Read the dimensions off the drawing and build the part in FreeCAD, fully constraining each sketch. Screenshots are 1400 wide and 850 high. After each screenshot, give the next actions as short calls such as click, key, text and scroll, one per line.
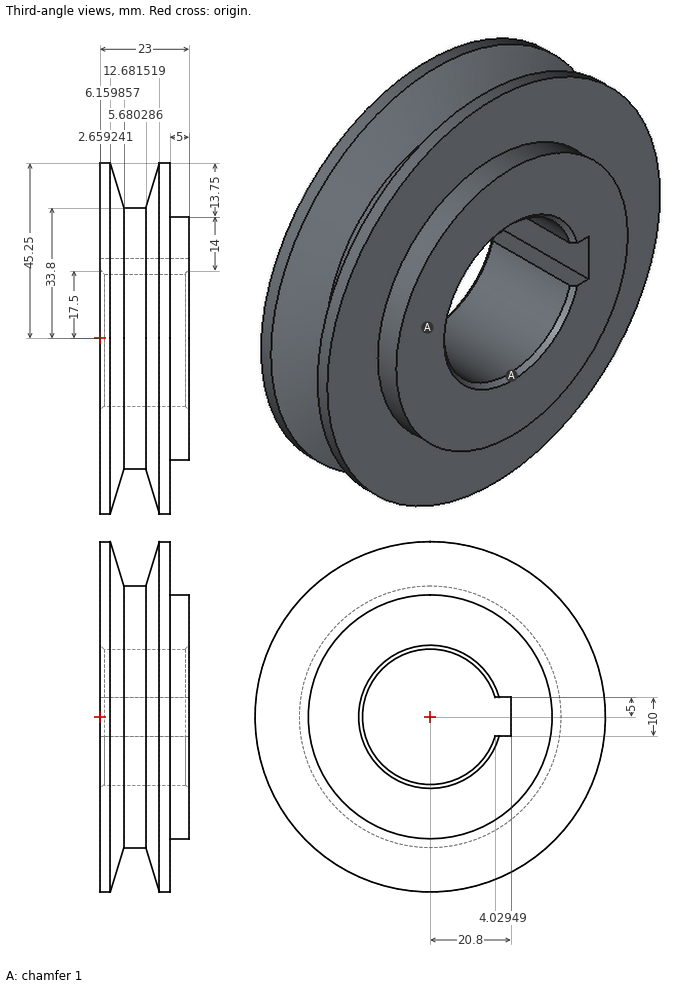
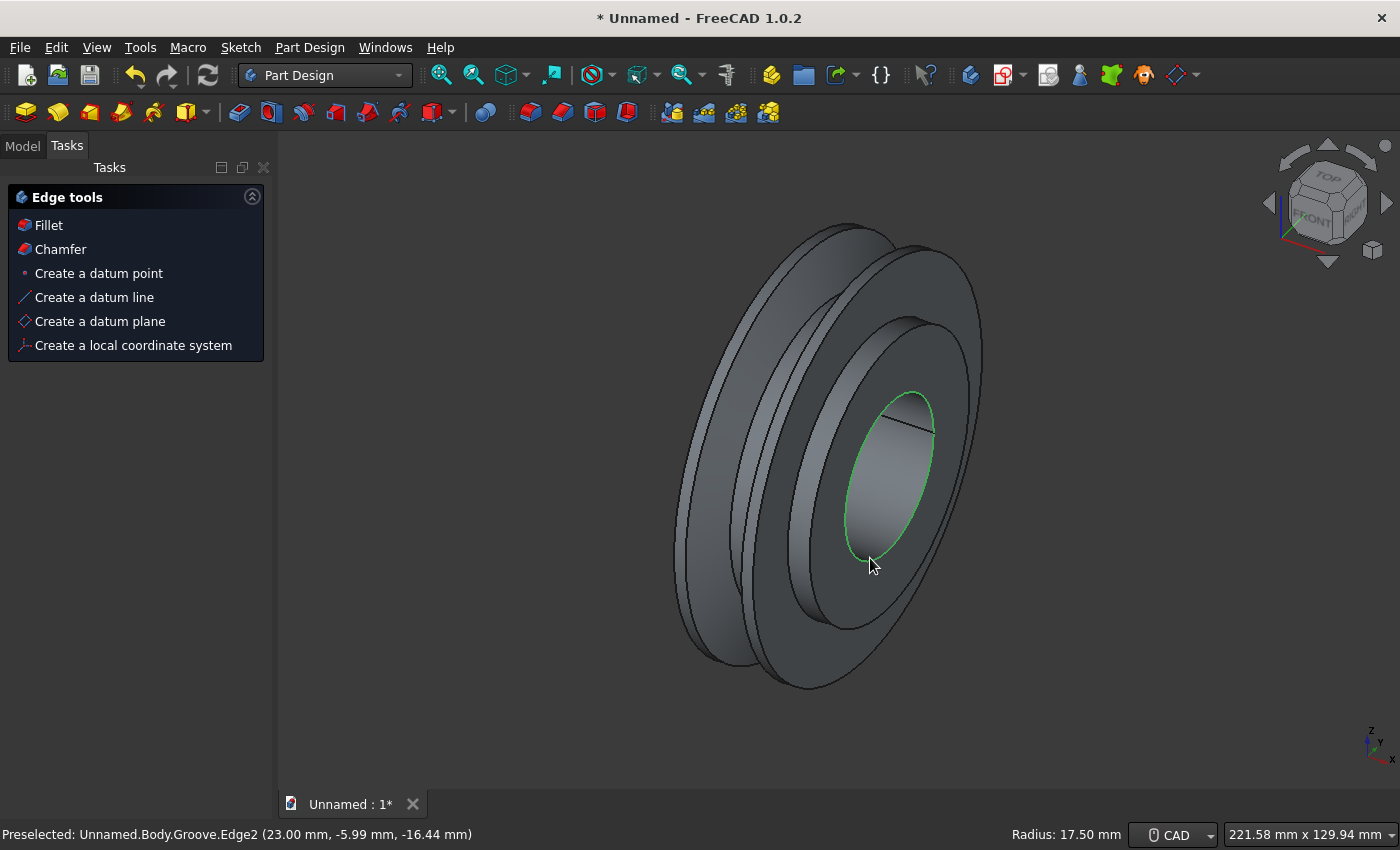
key(0)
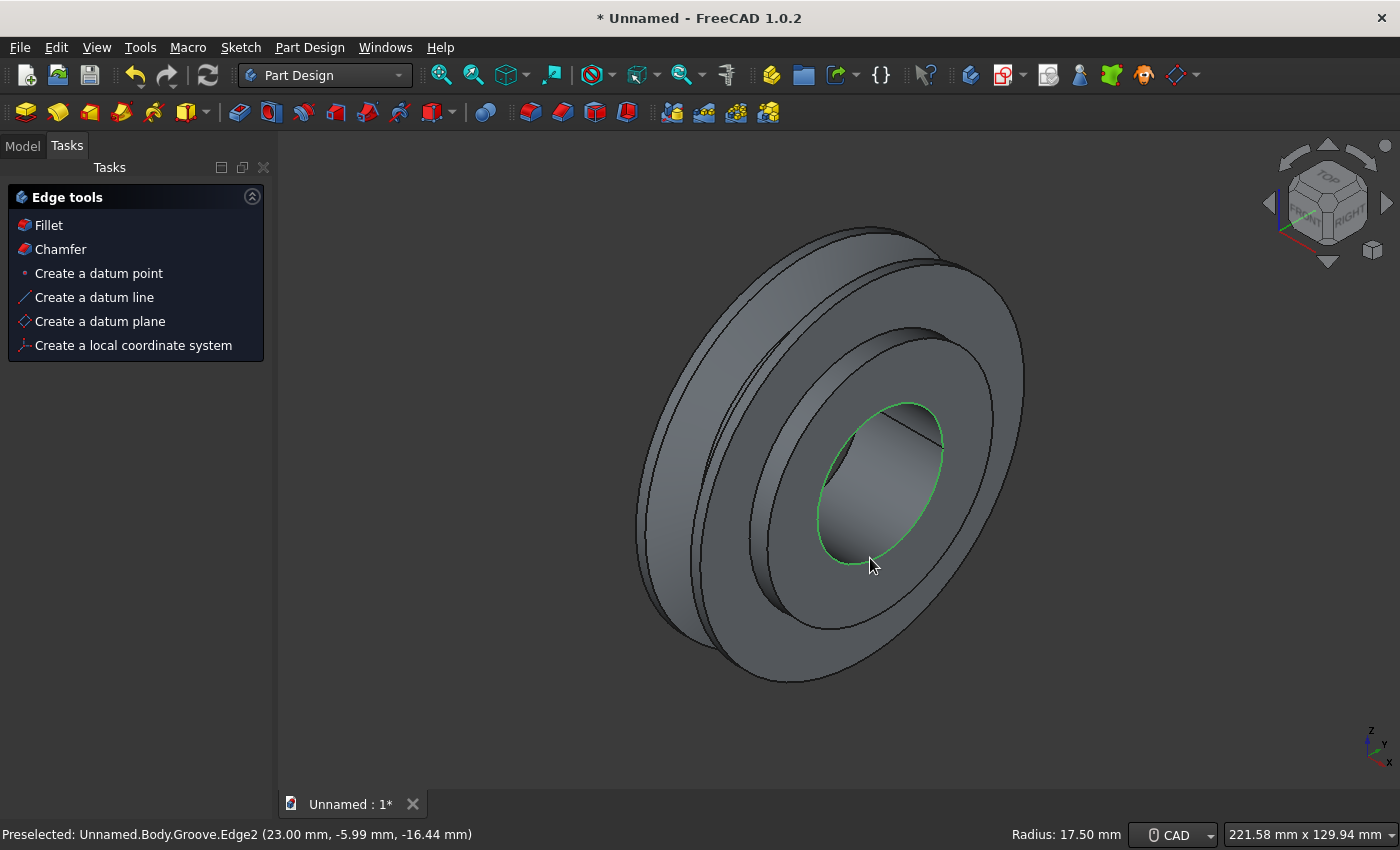
key(2)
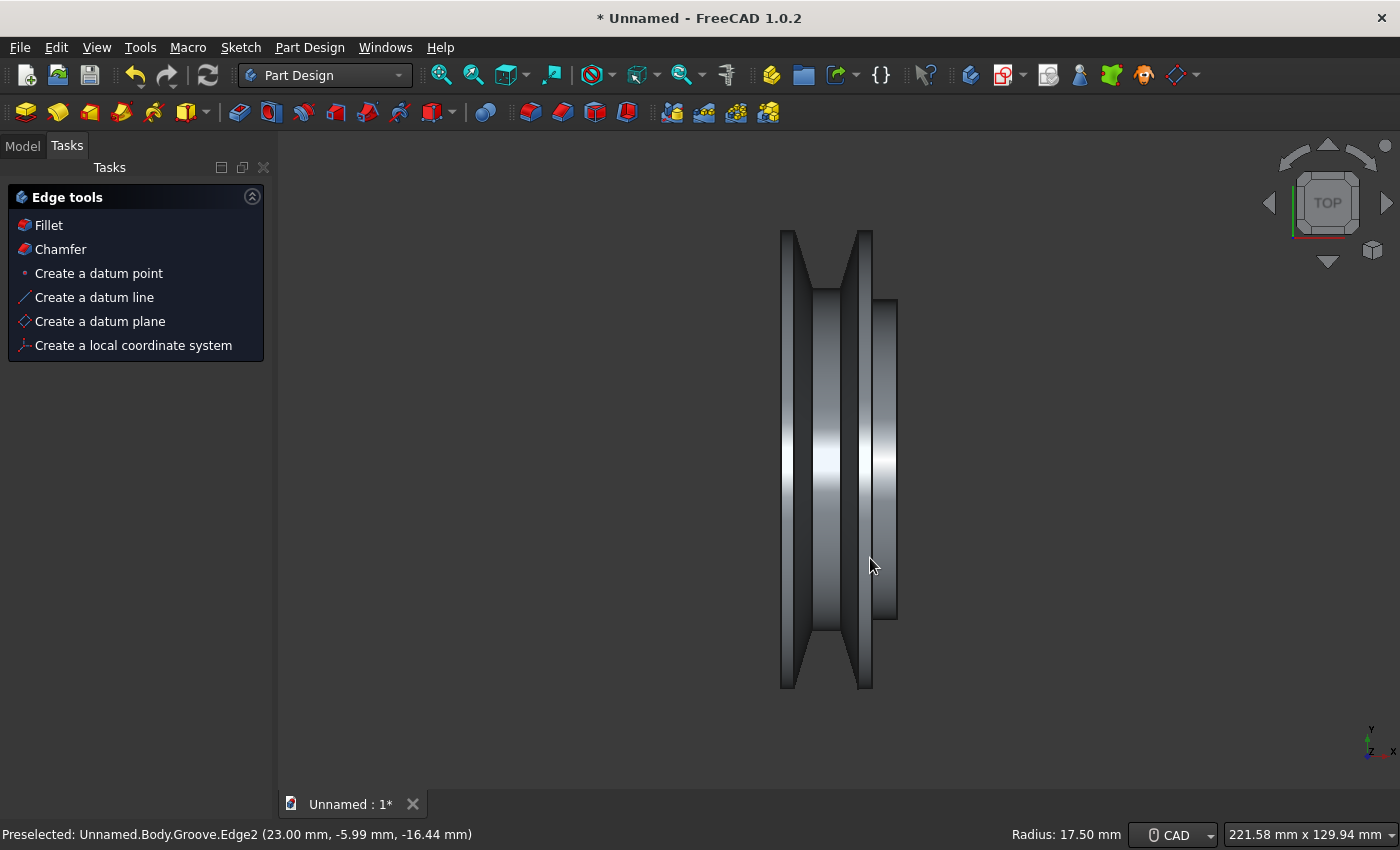
key(1)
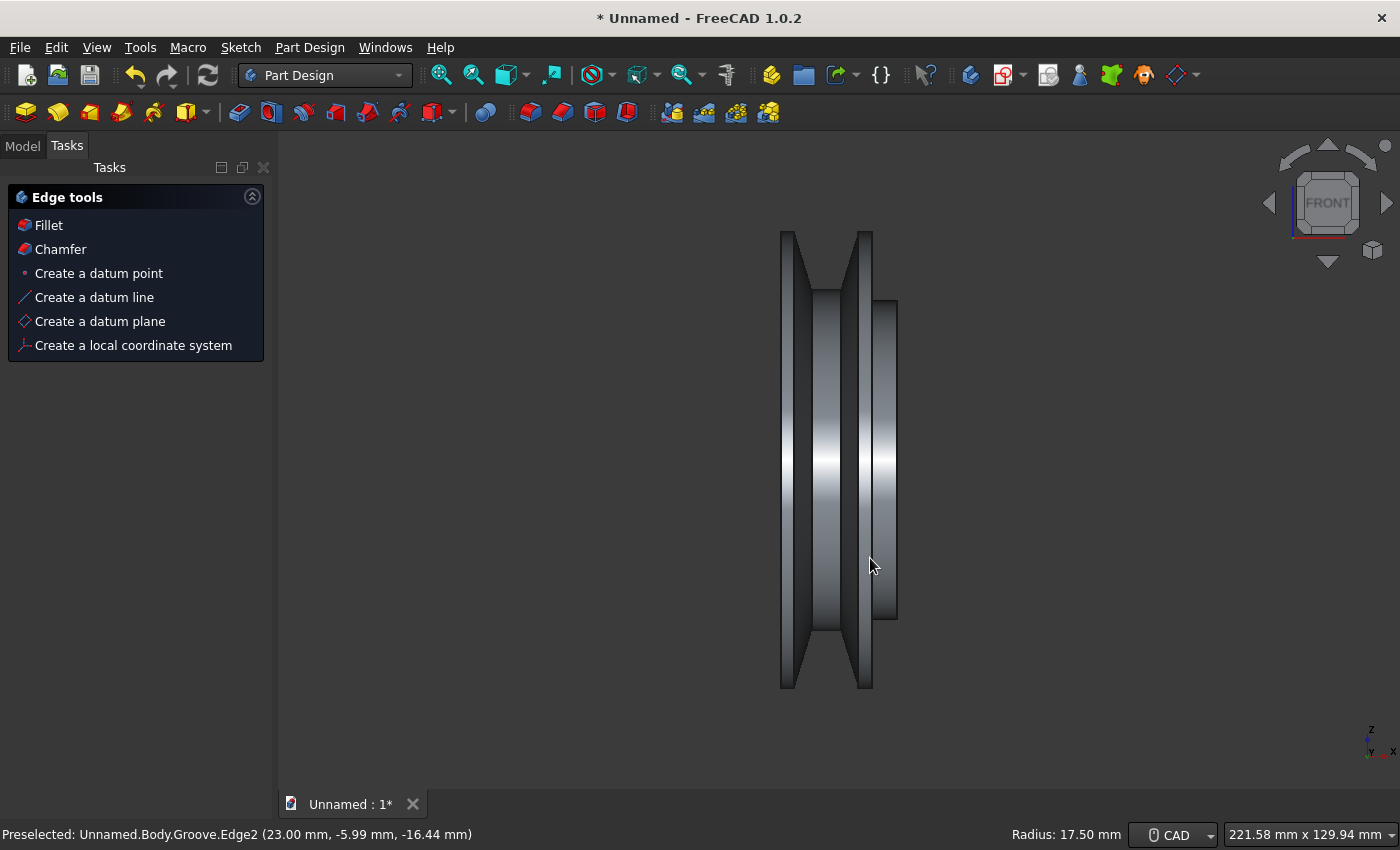
key(3)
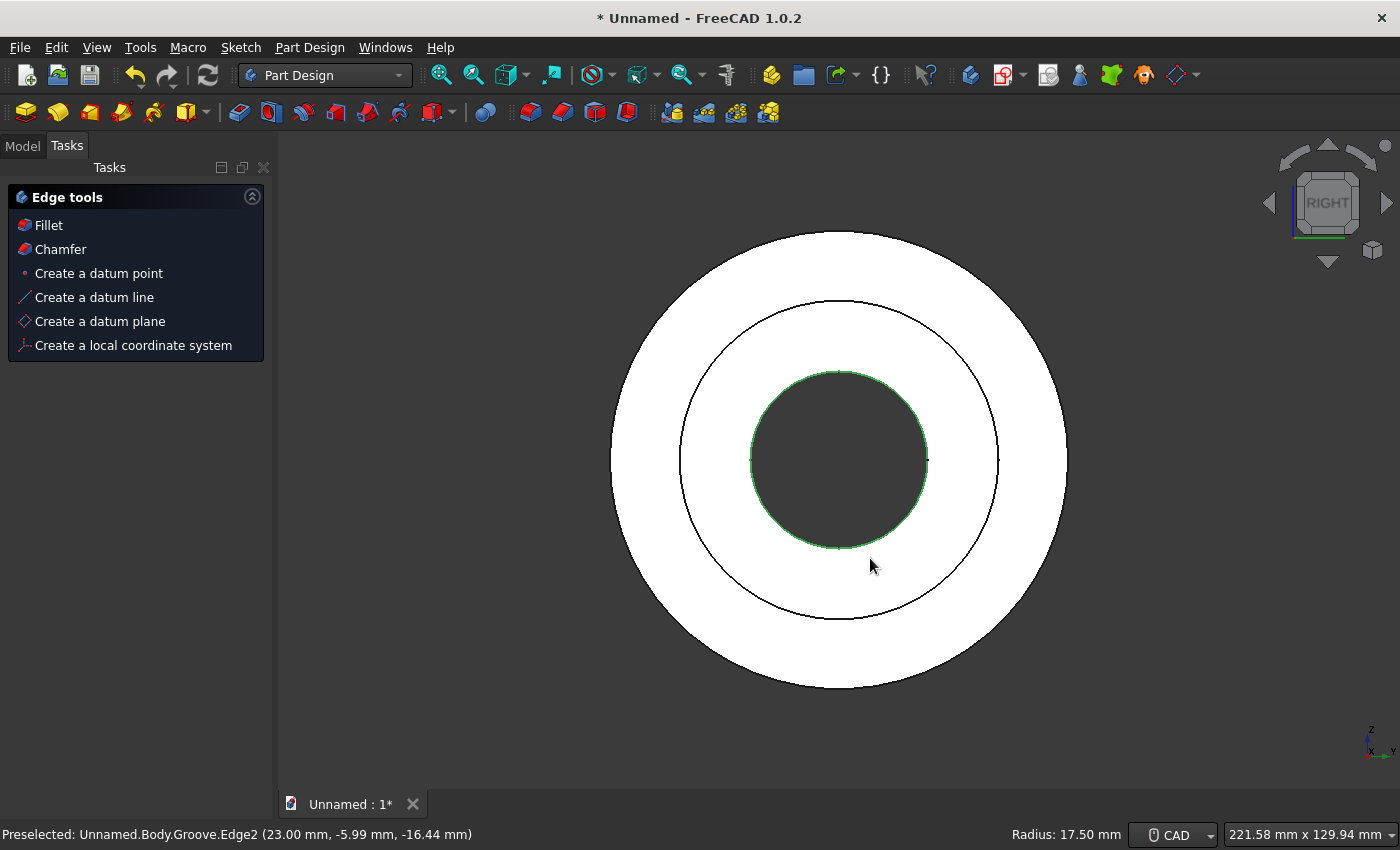
key(5)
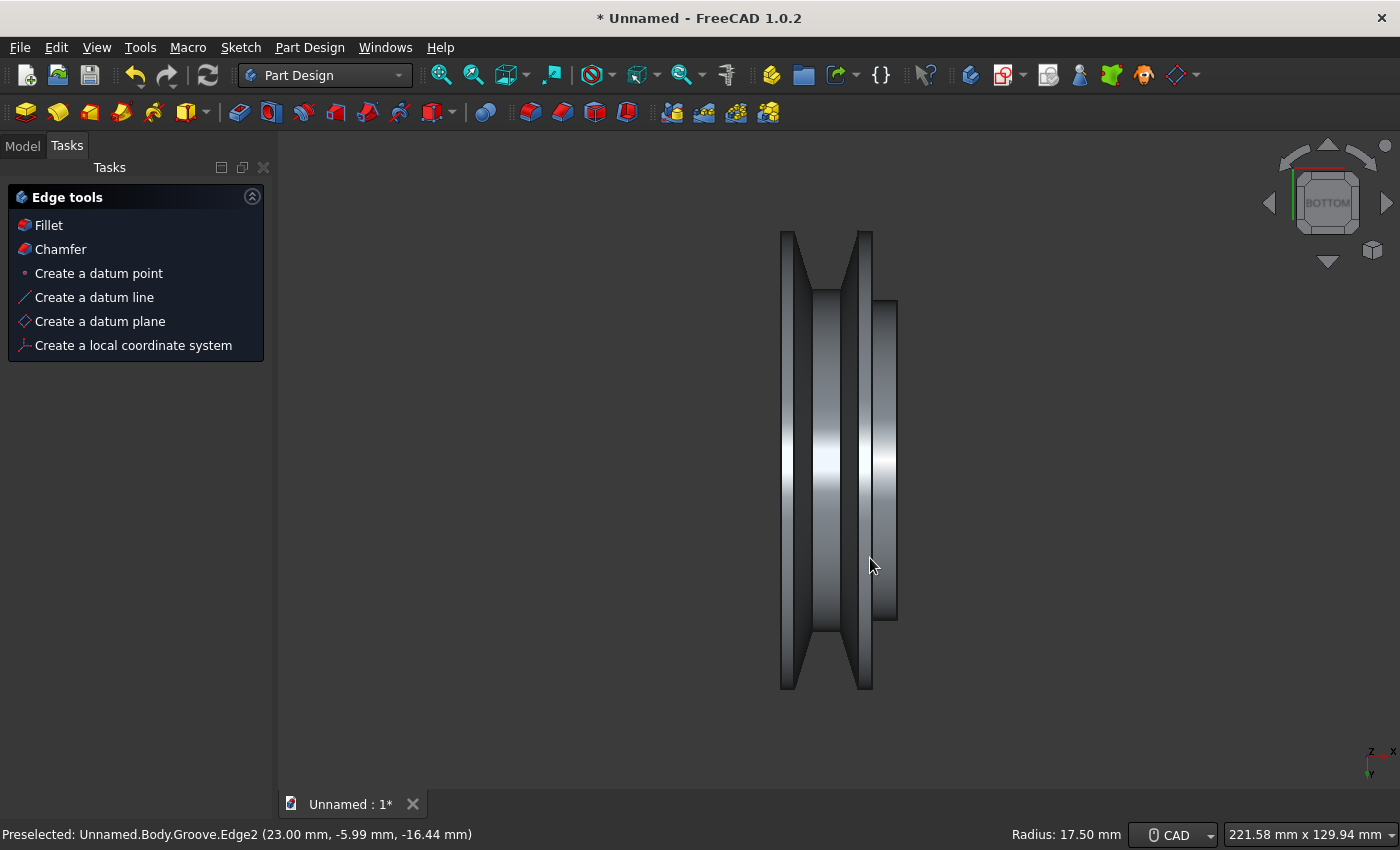
key(4)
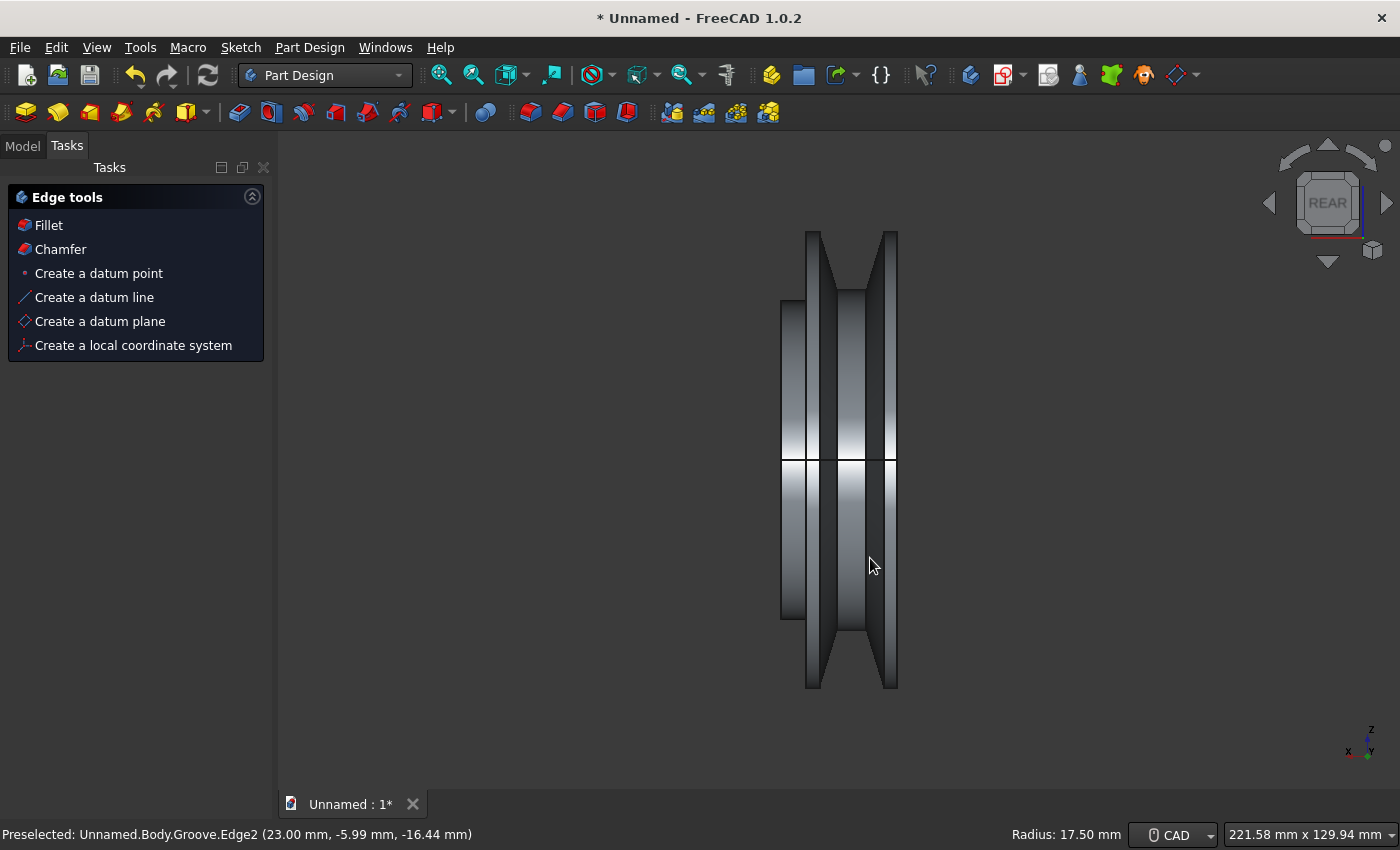
key(6)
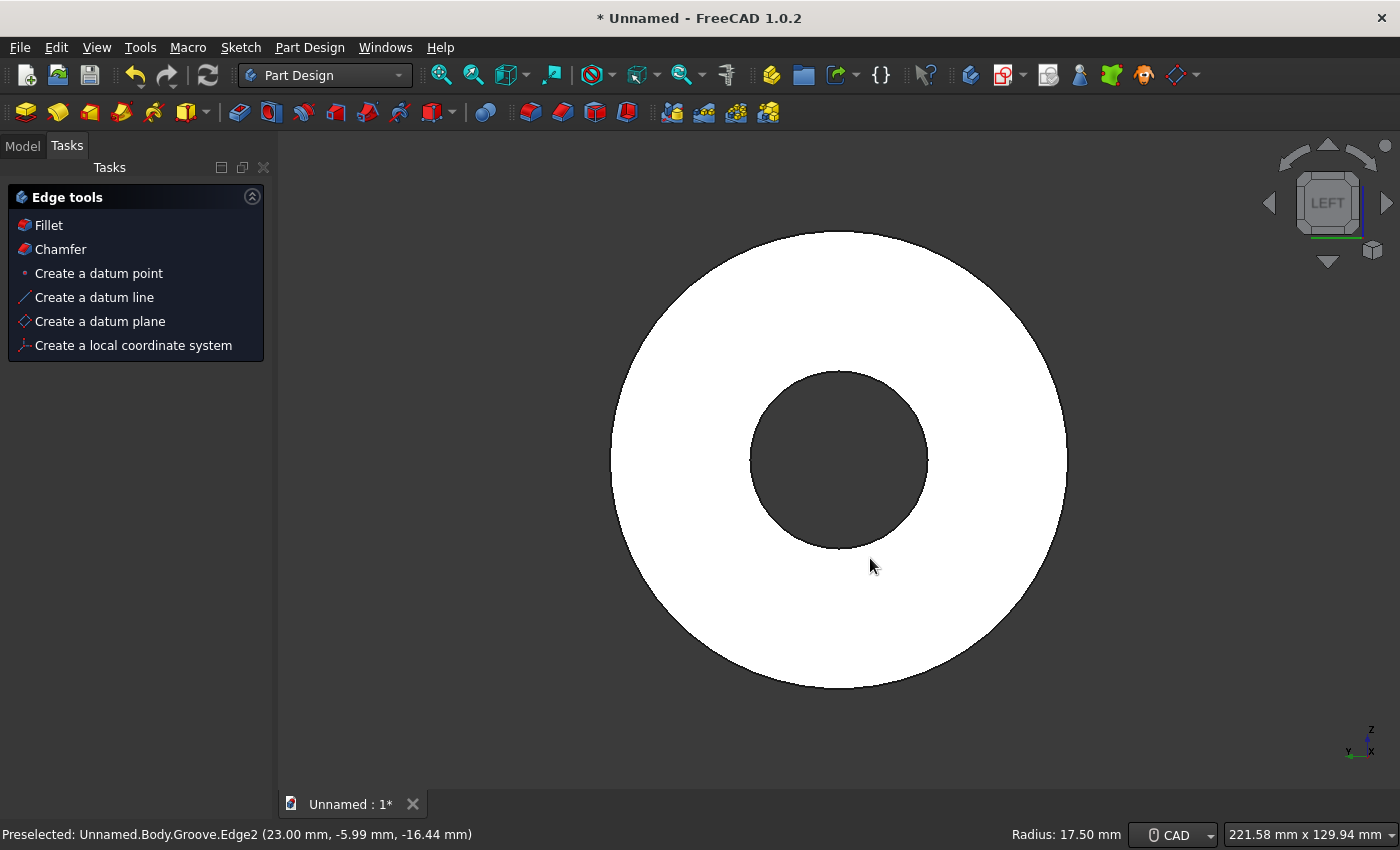
click(928, 459, ctrl)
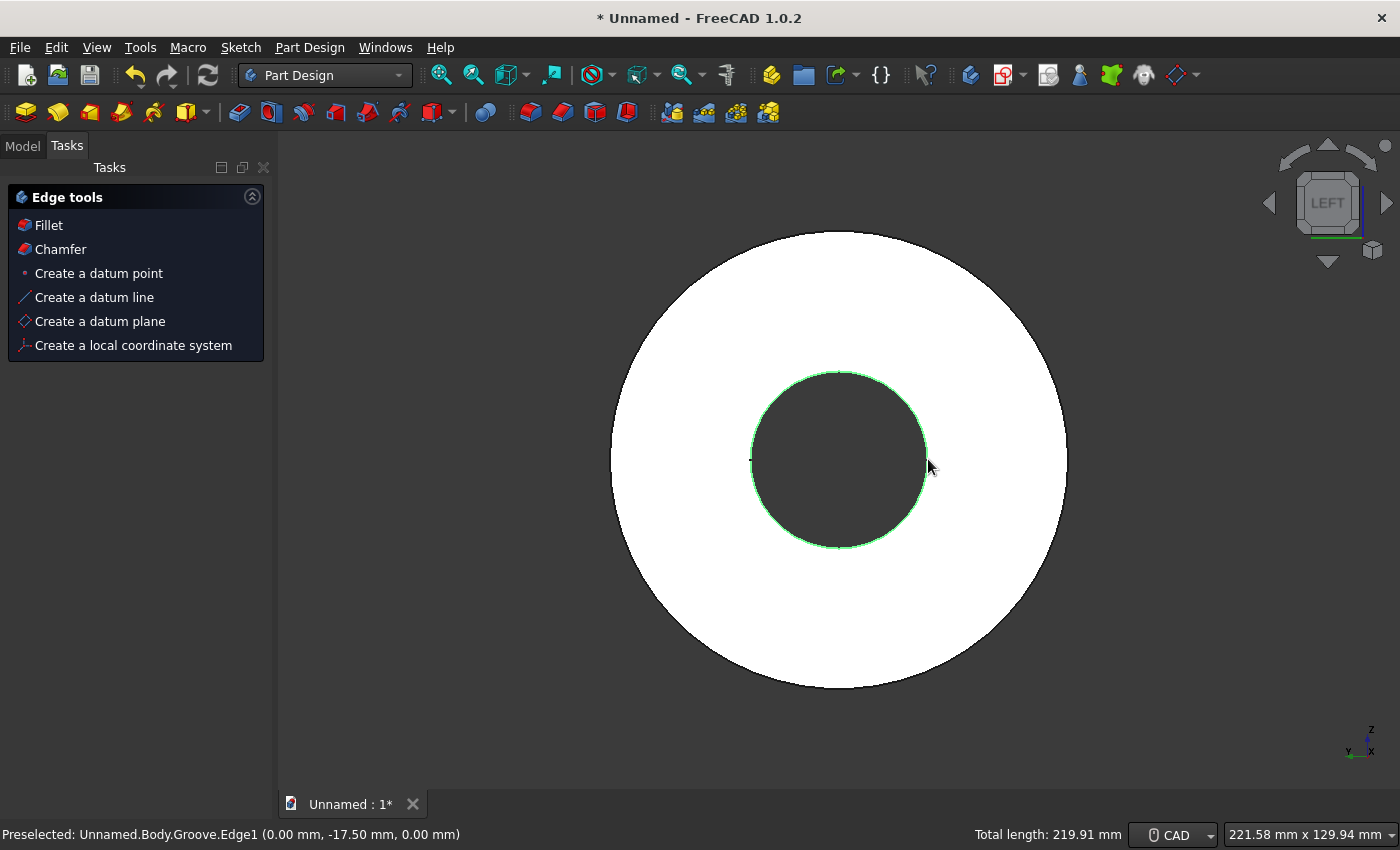
click(564, 112)